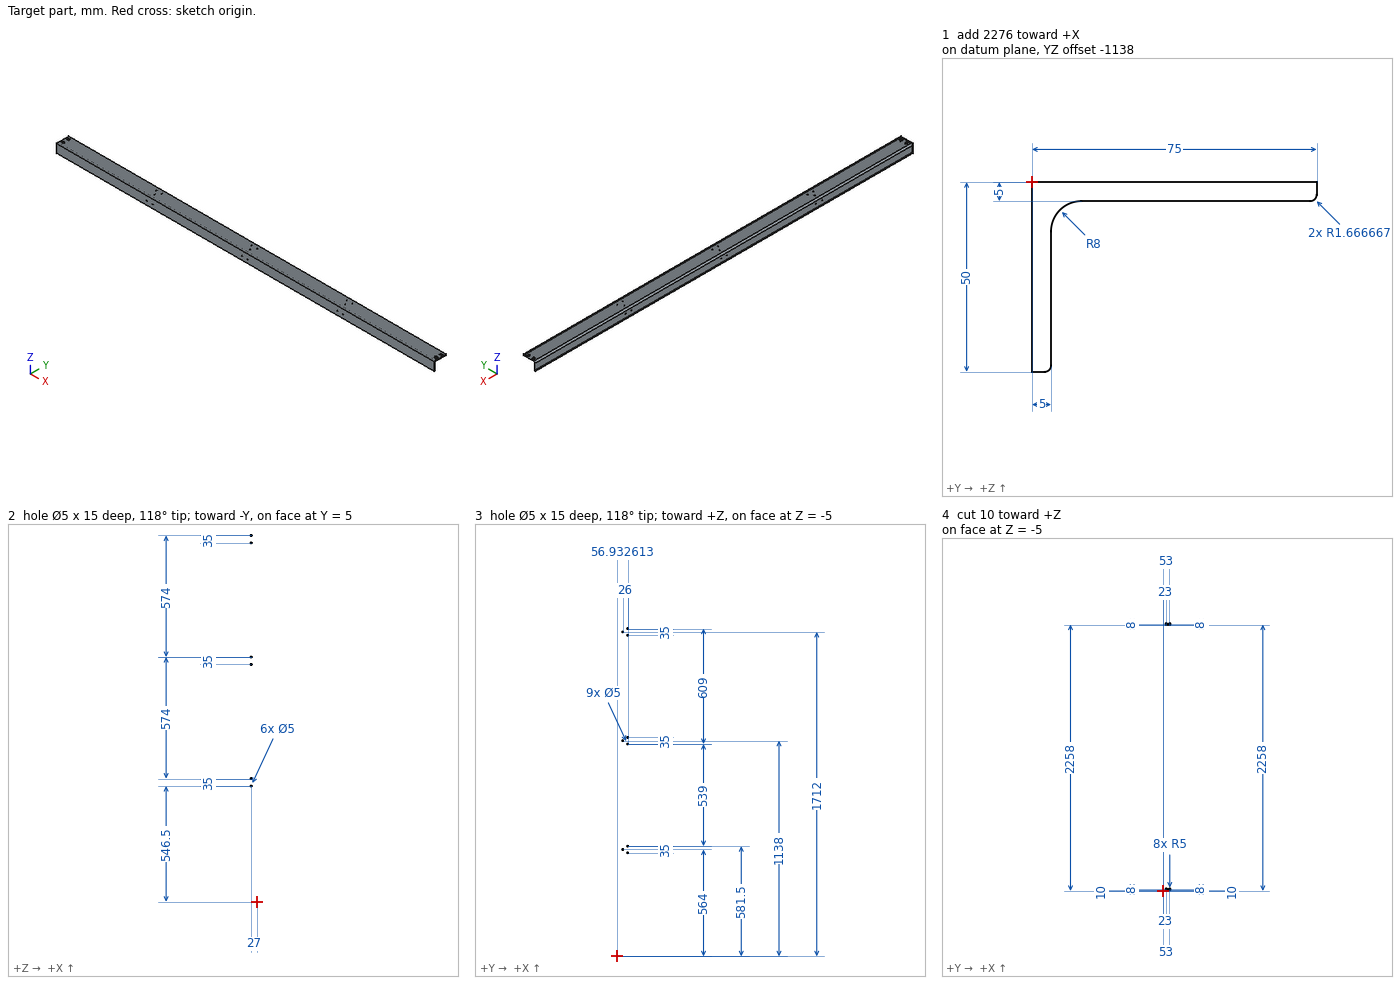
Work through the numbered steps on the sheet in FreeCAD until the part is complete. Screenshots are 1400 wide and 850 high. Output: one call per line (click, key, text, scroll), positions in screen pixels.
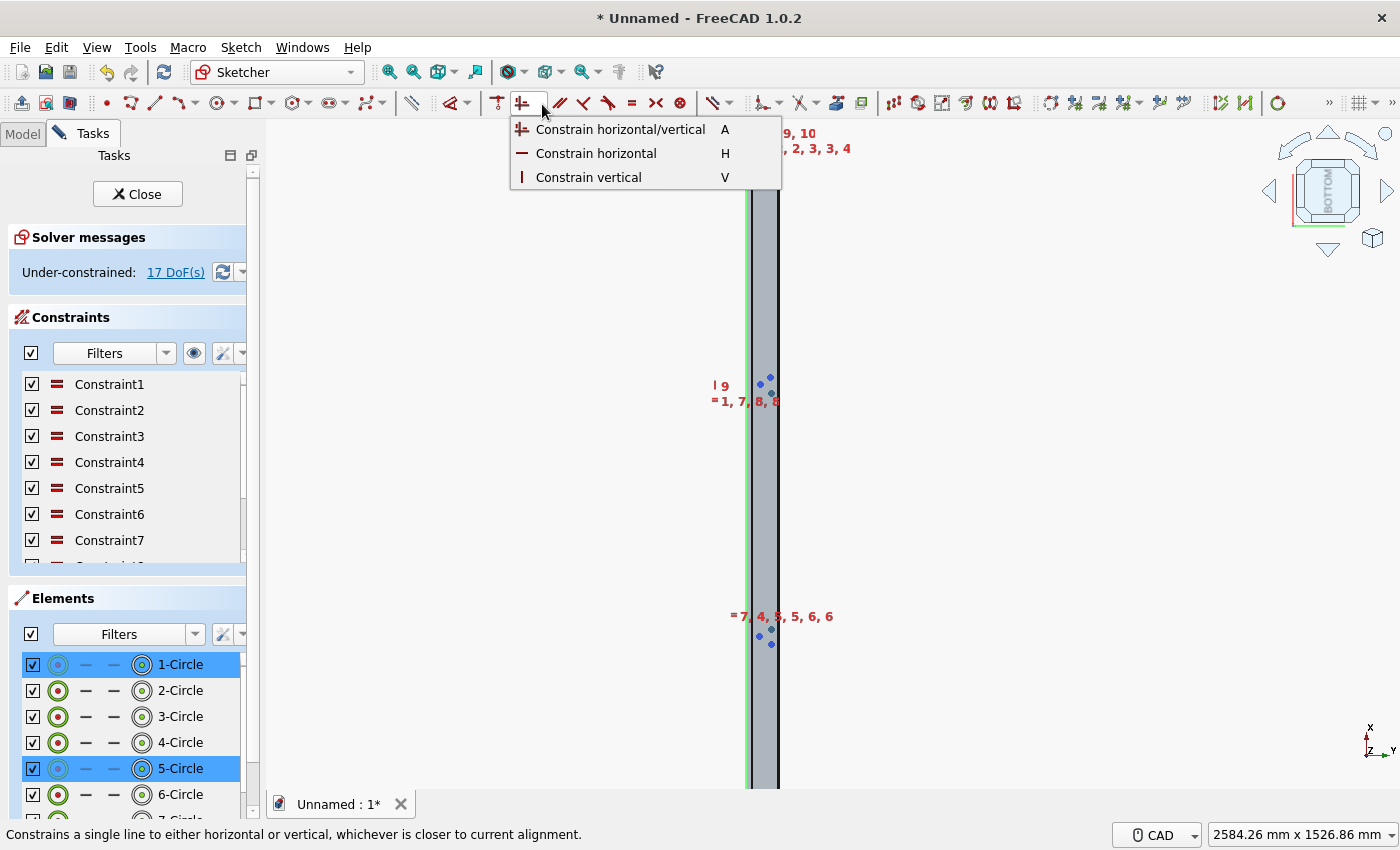
click(646, 177)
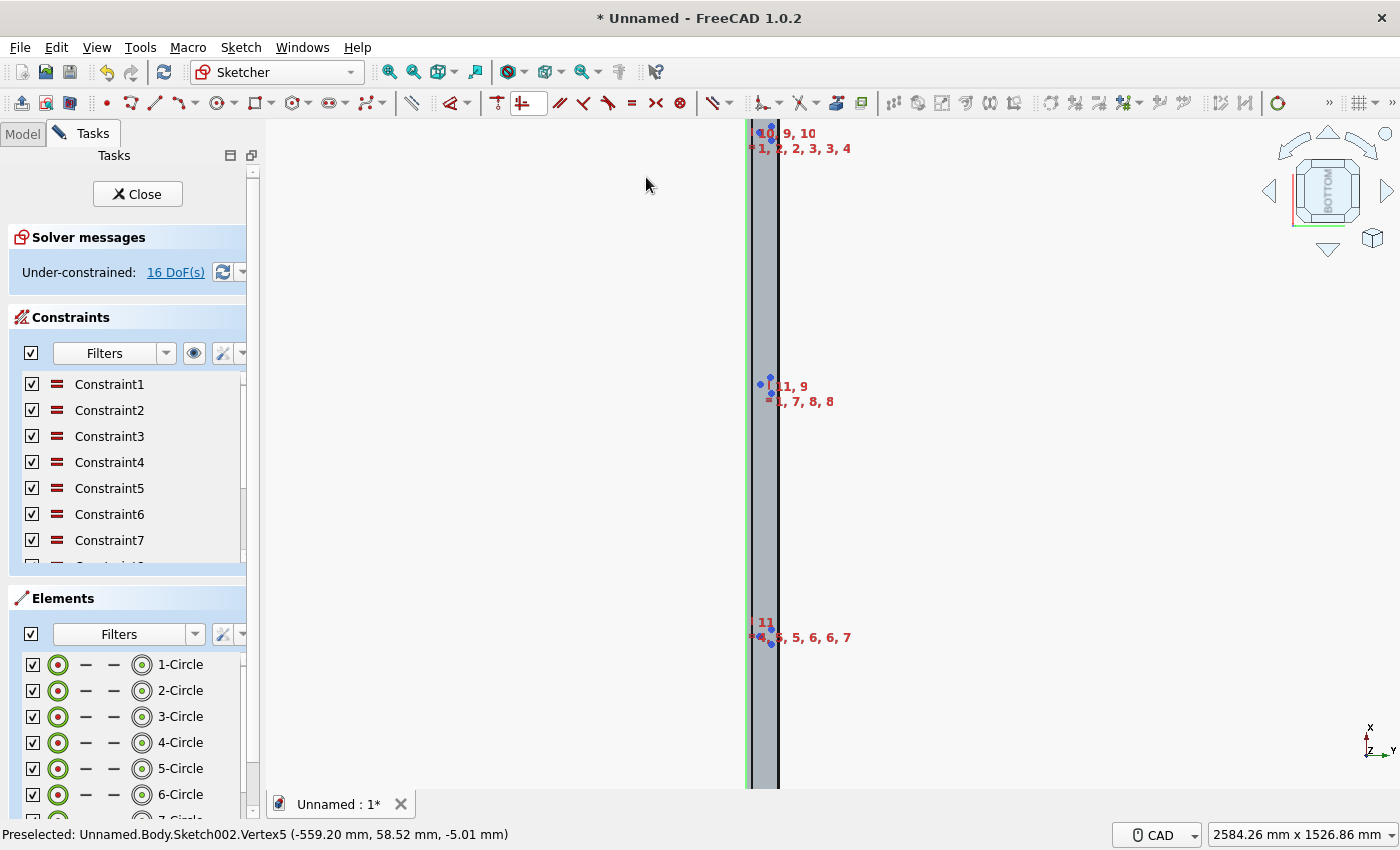
scroll(771, 629, up, 4)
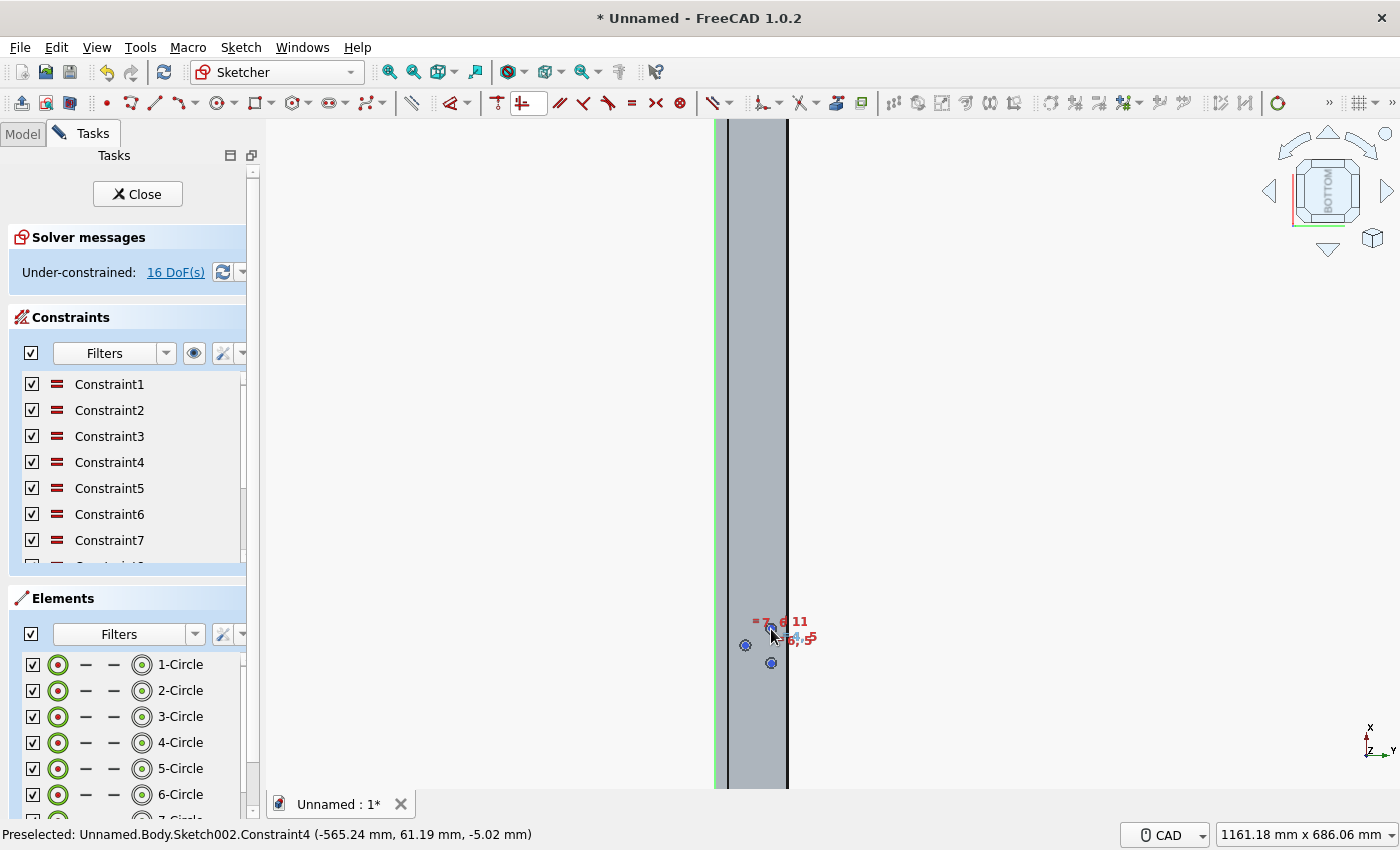
click(771, 629)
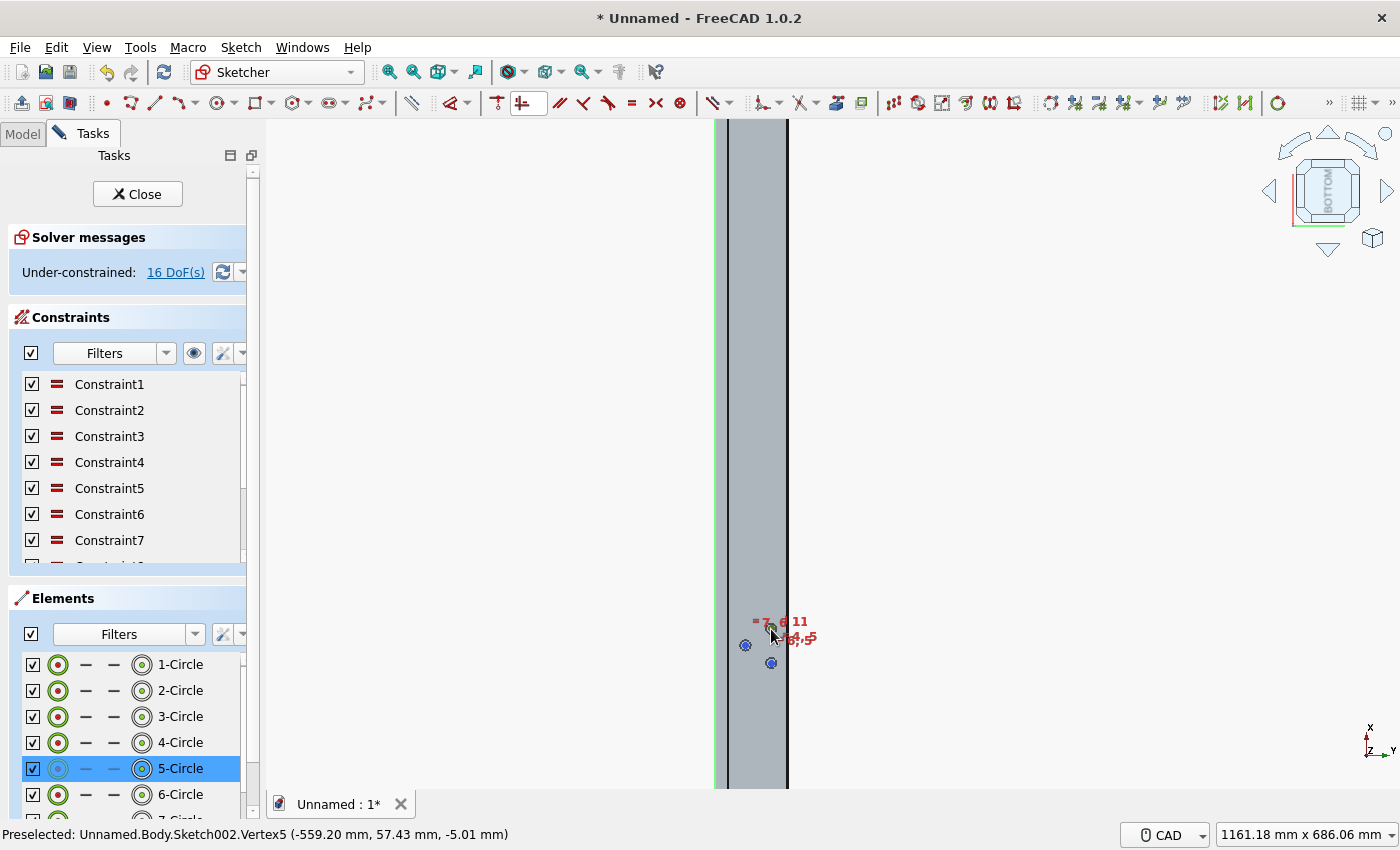
click(771, 663)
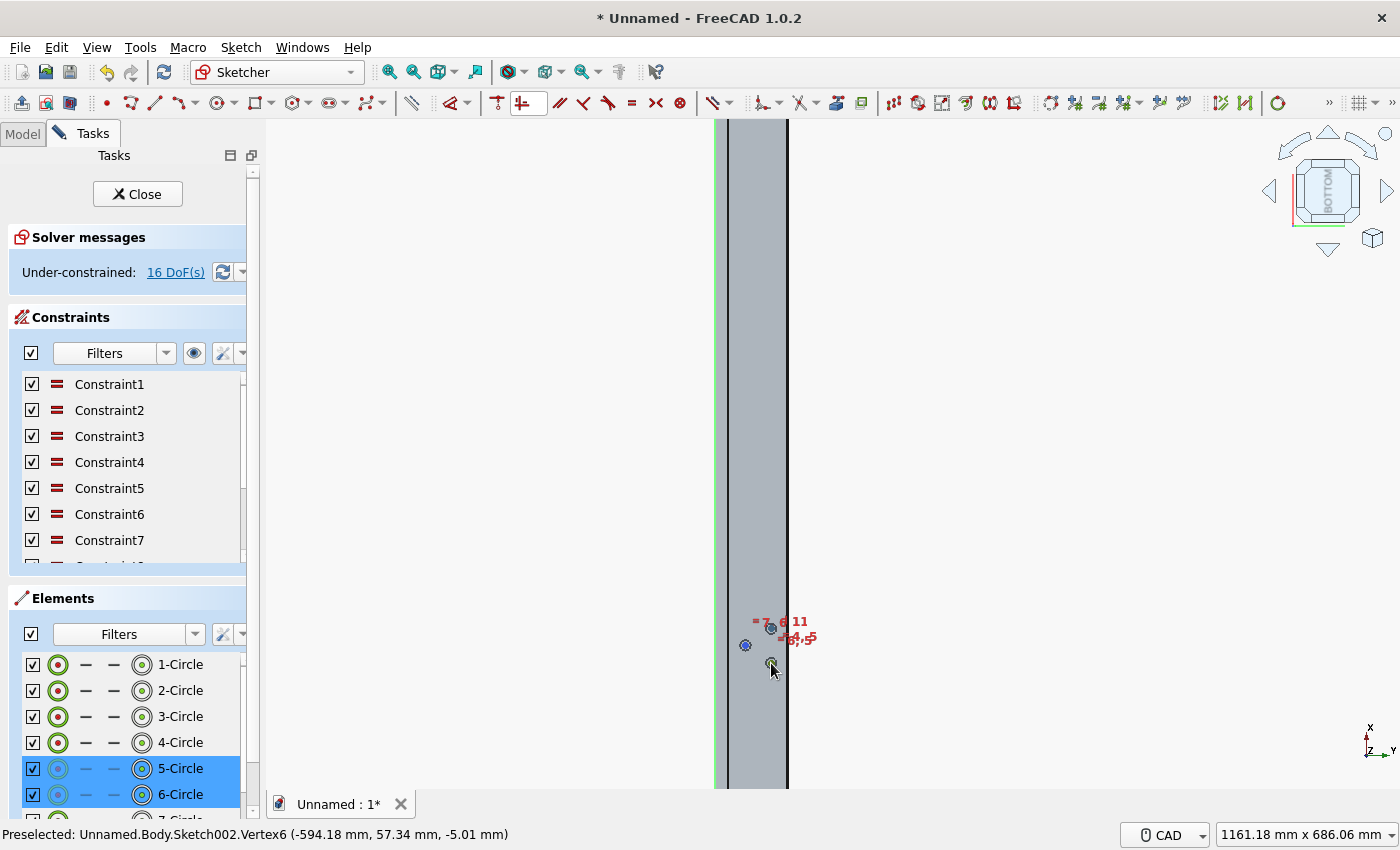
click(542, 104)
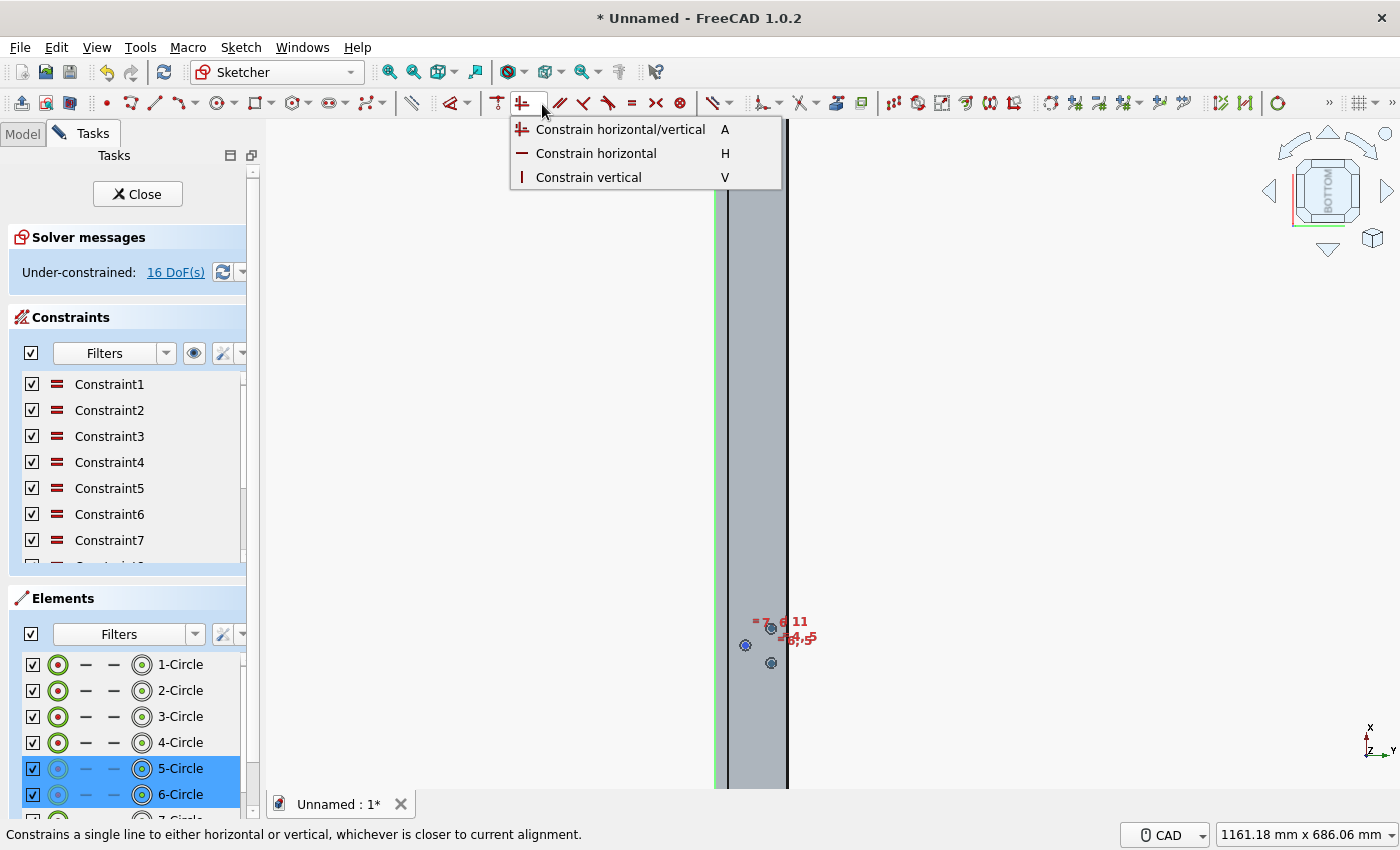
click(646, 177)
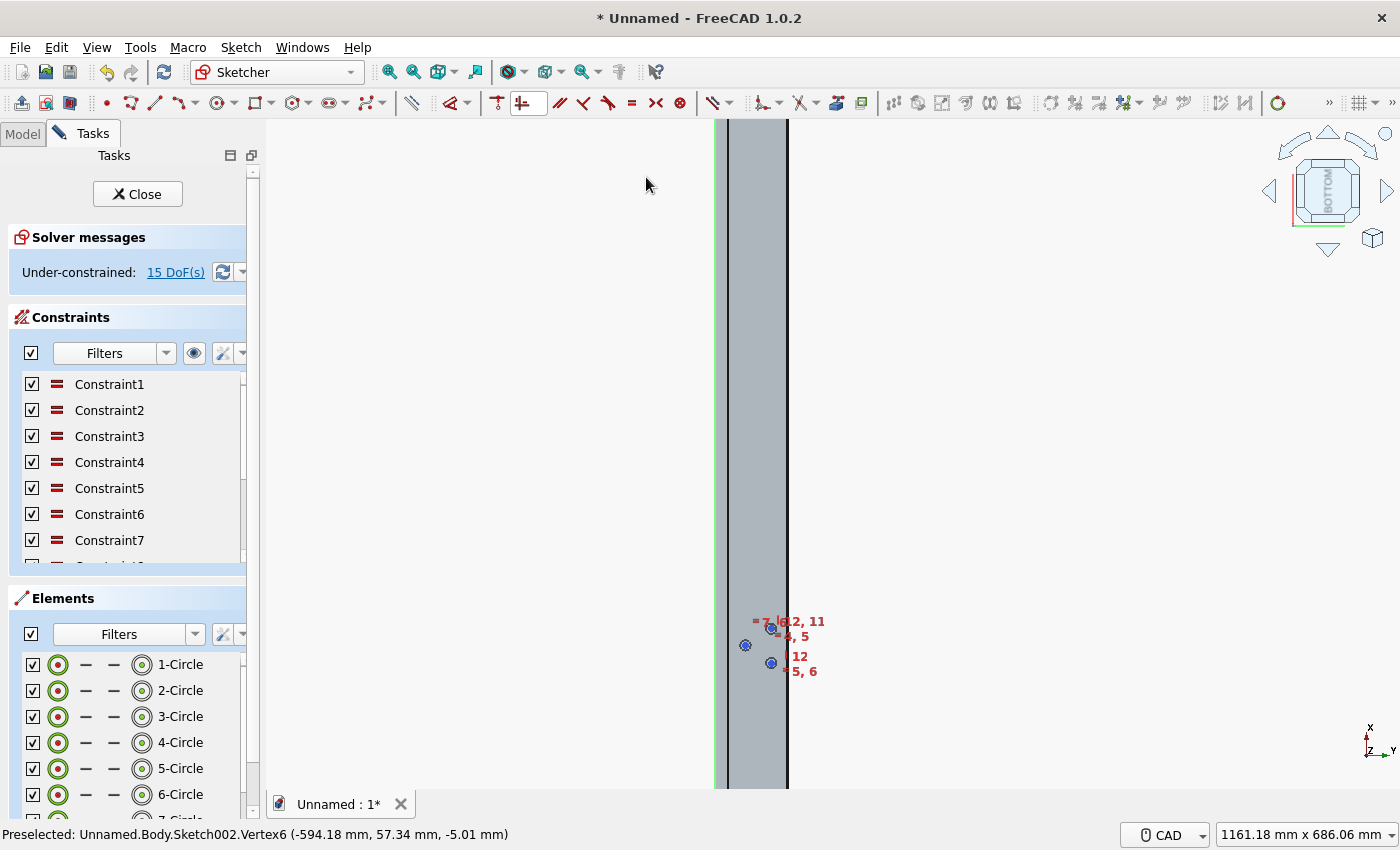
scroll(771, 489, down, 7)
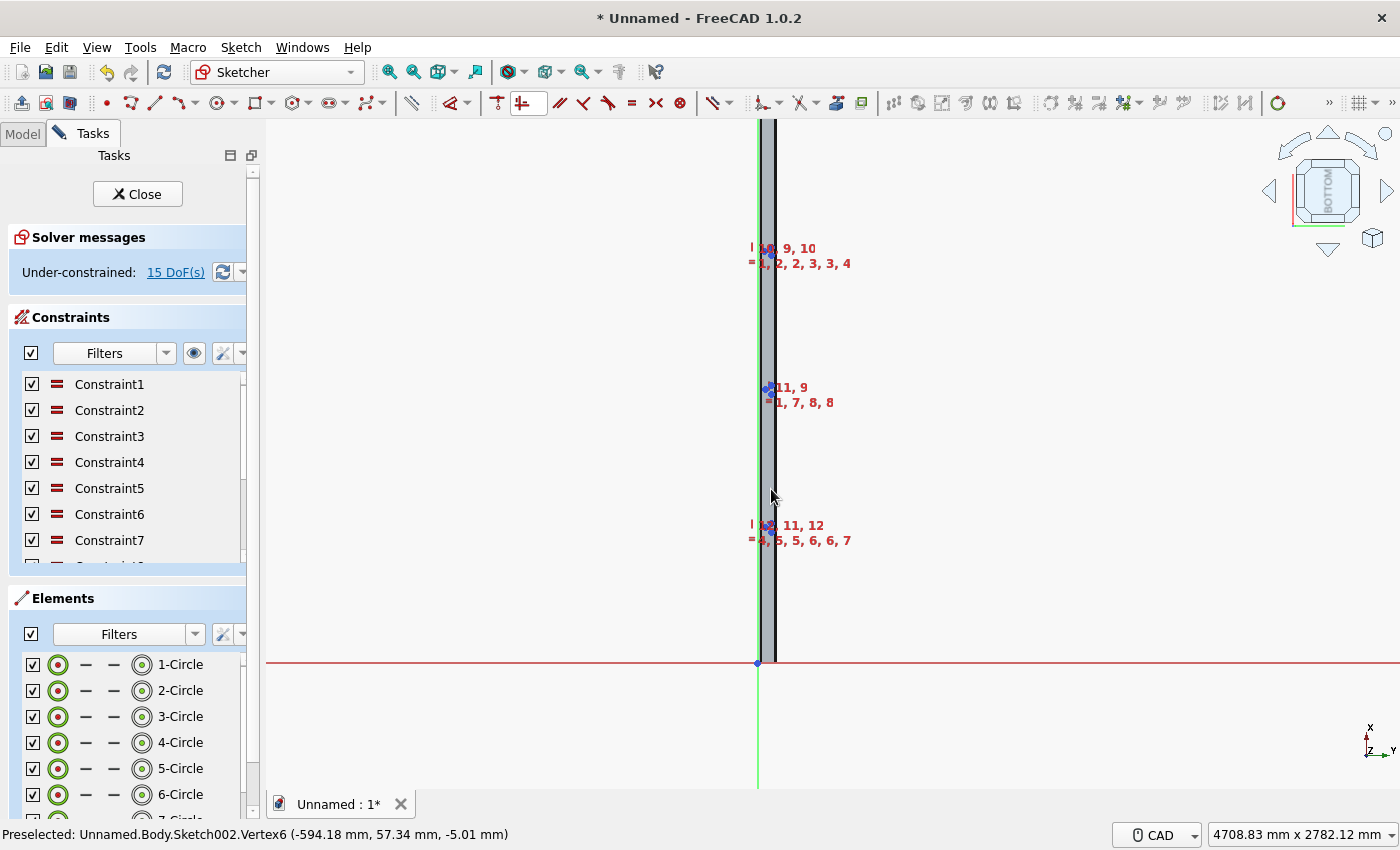
scroll(765, 251, up, 3)